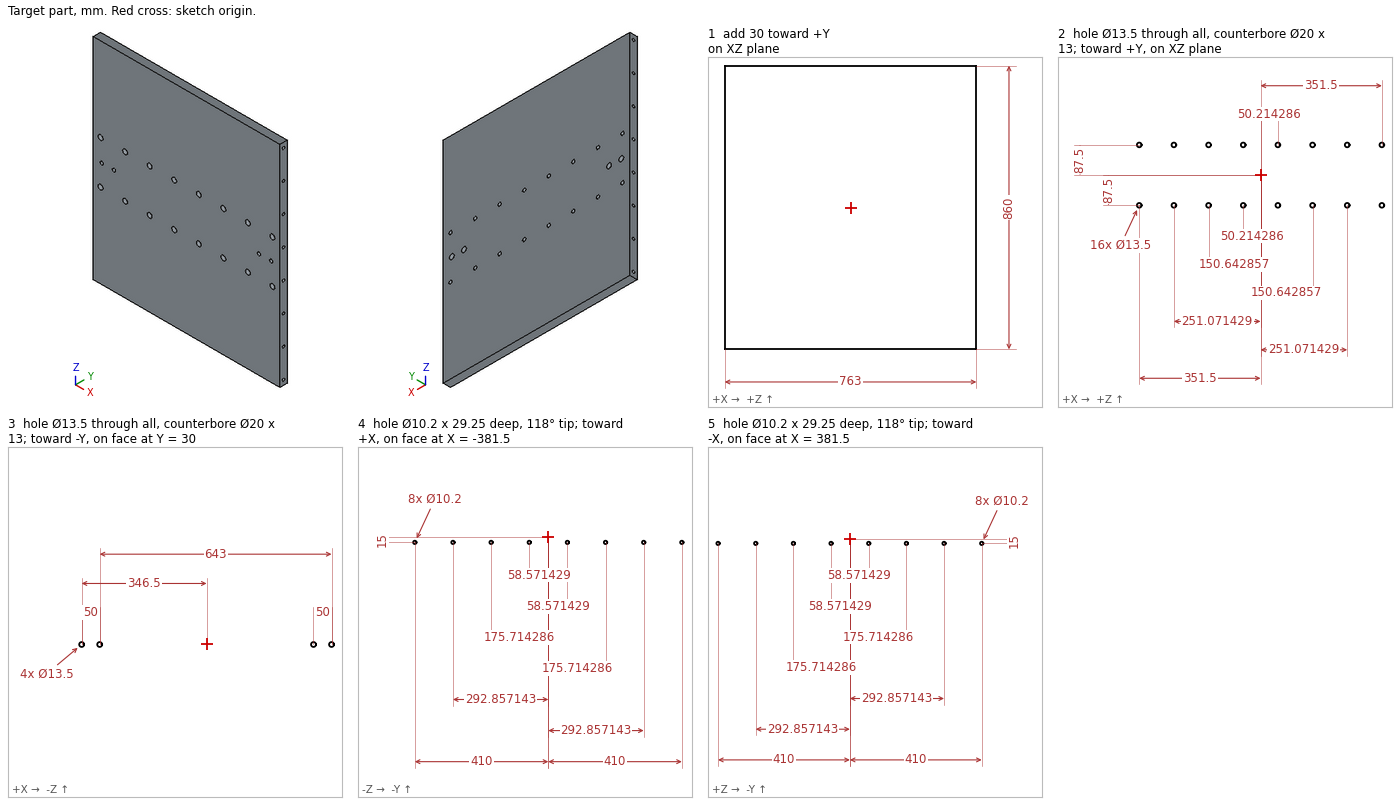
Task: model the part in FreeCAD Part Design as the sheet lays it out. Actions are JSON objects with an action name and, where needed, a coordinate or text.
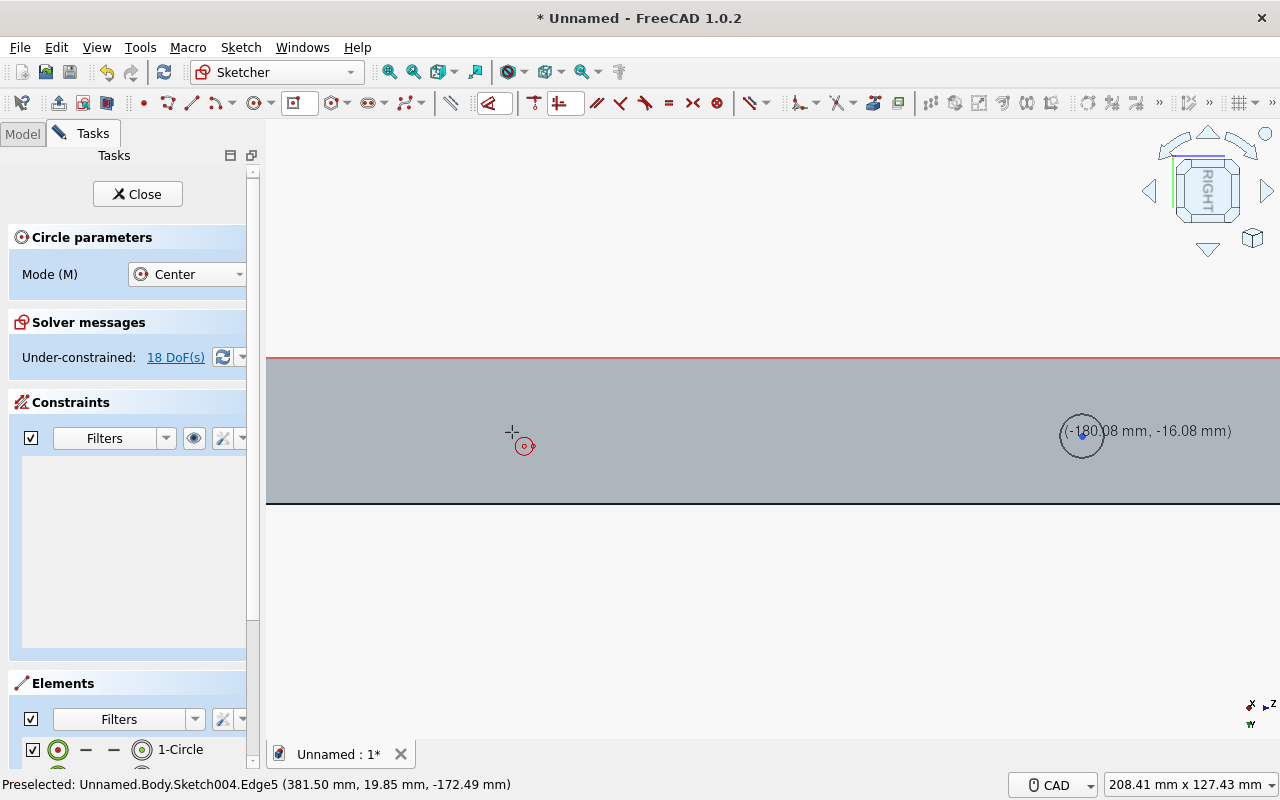
{"action": "scroll", "coordinate": [512, 432], "scroll_direction": "down", "scroll_amount": 10}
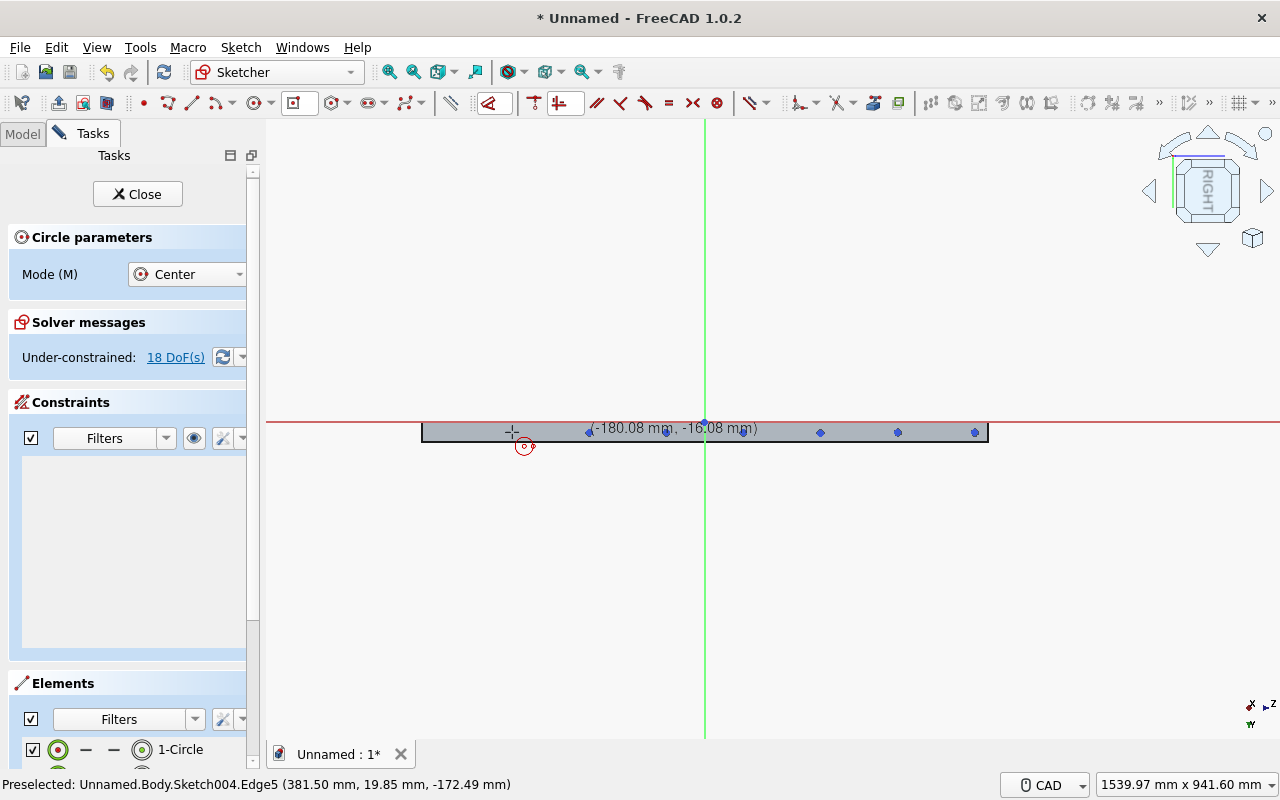
{"action": "scroll", "coordinate": [512, 432], "scroll_direction": "up", "scroll_amount": 3}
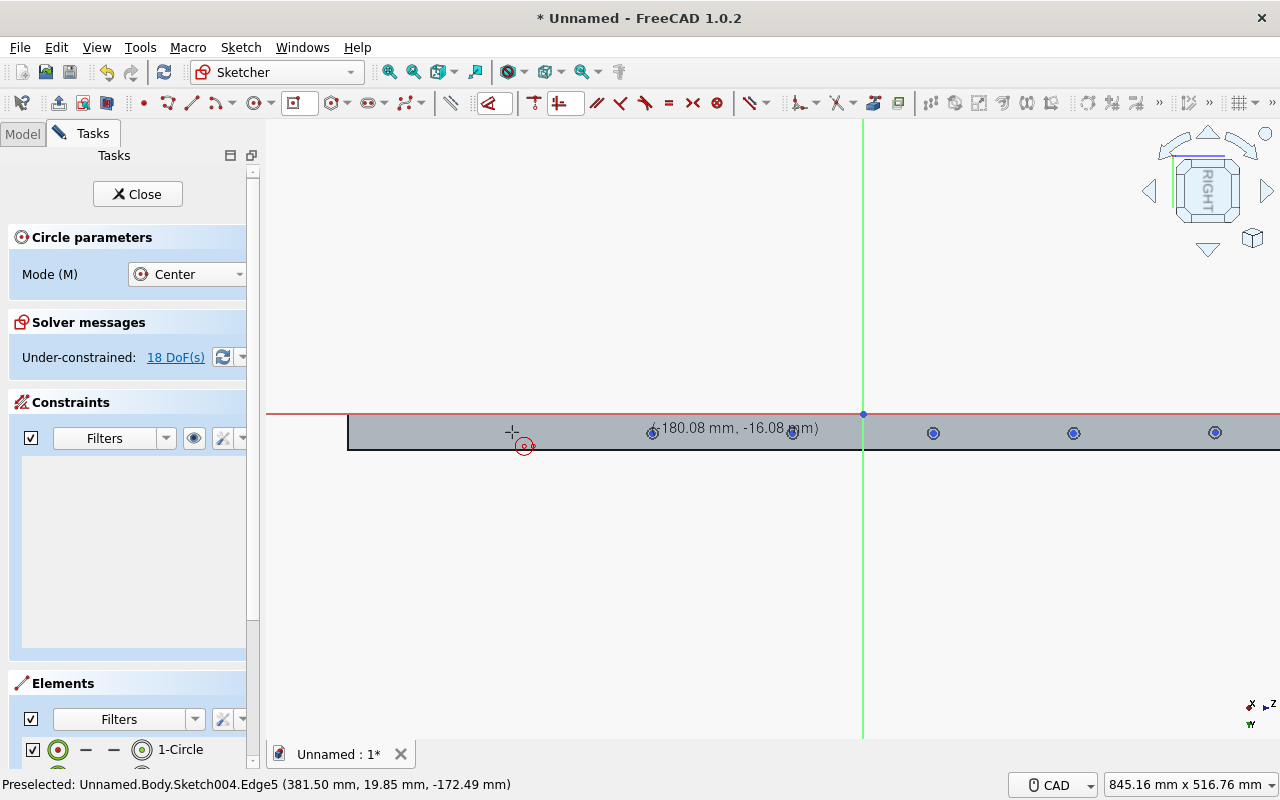
{"action": "left_click", "coordinate": [512, 432]}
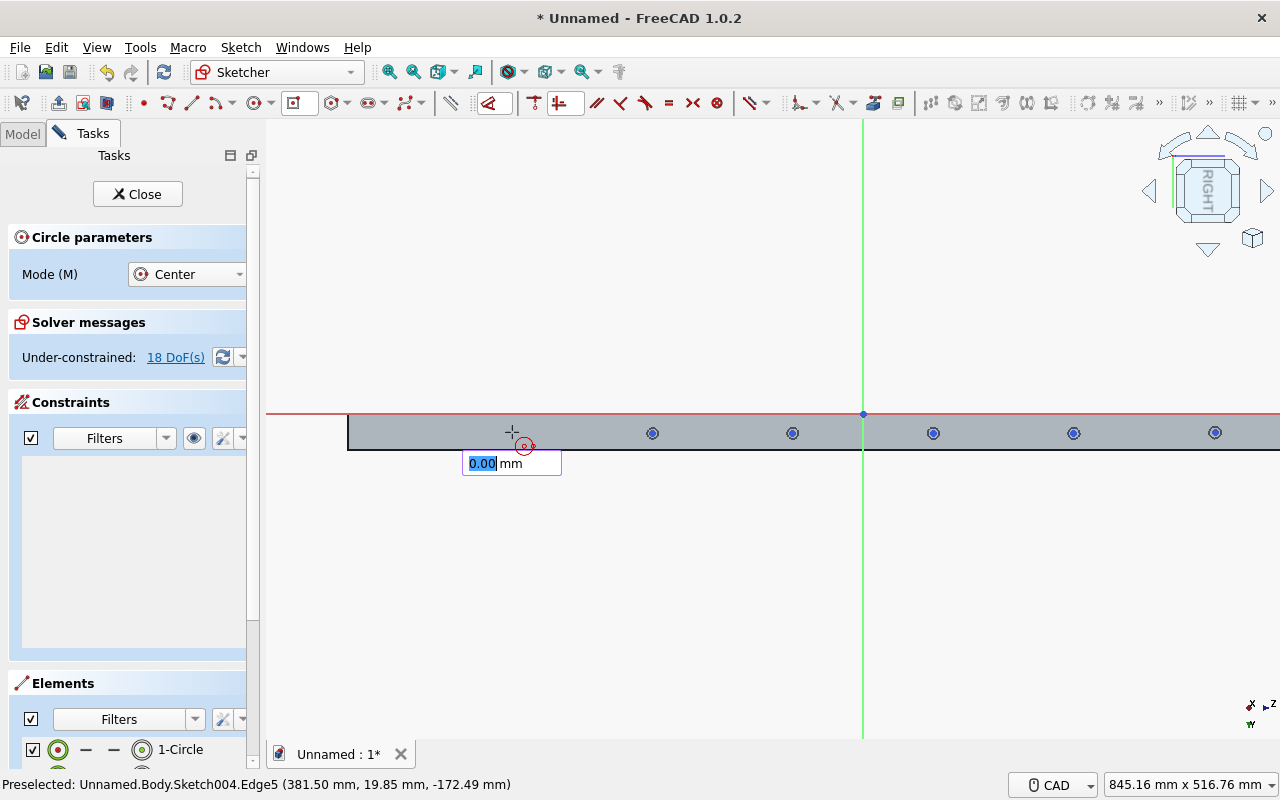
{"action": "scroll", "coordinate": [516, 436], "scroll_direction": "up", "scroll_amount": 5}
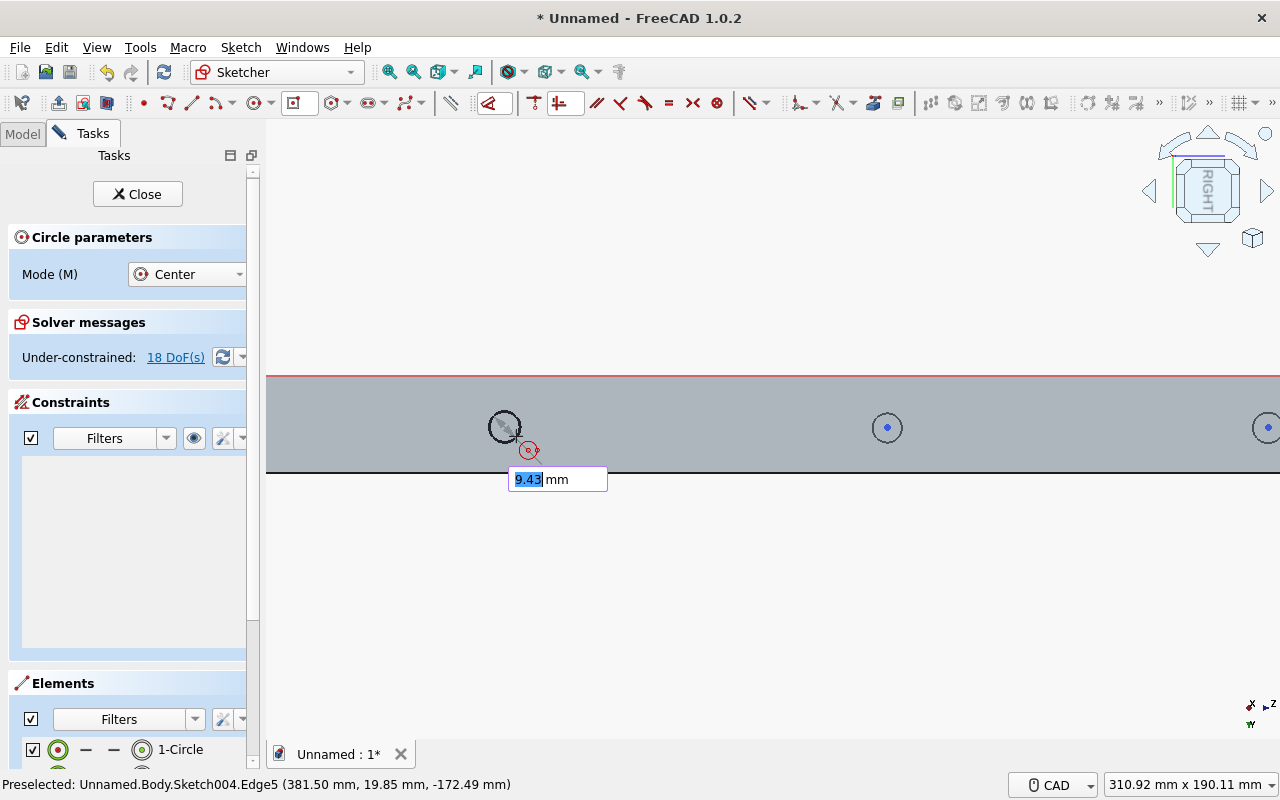
{"action": "left_click", "coordinate": [517, 436]}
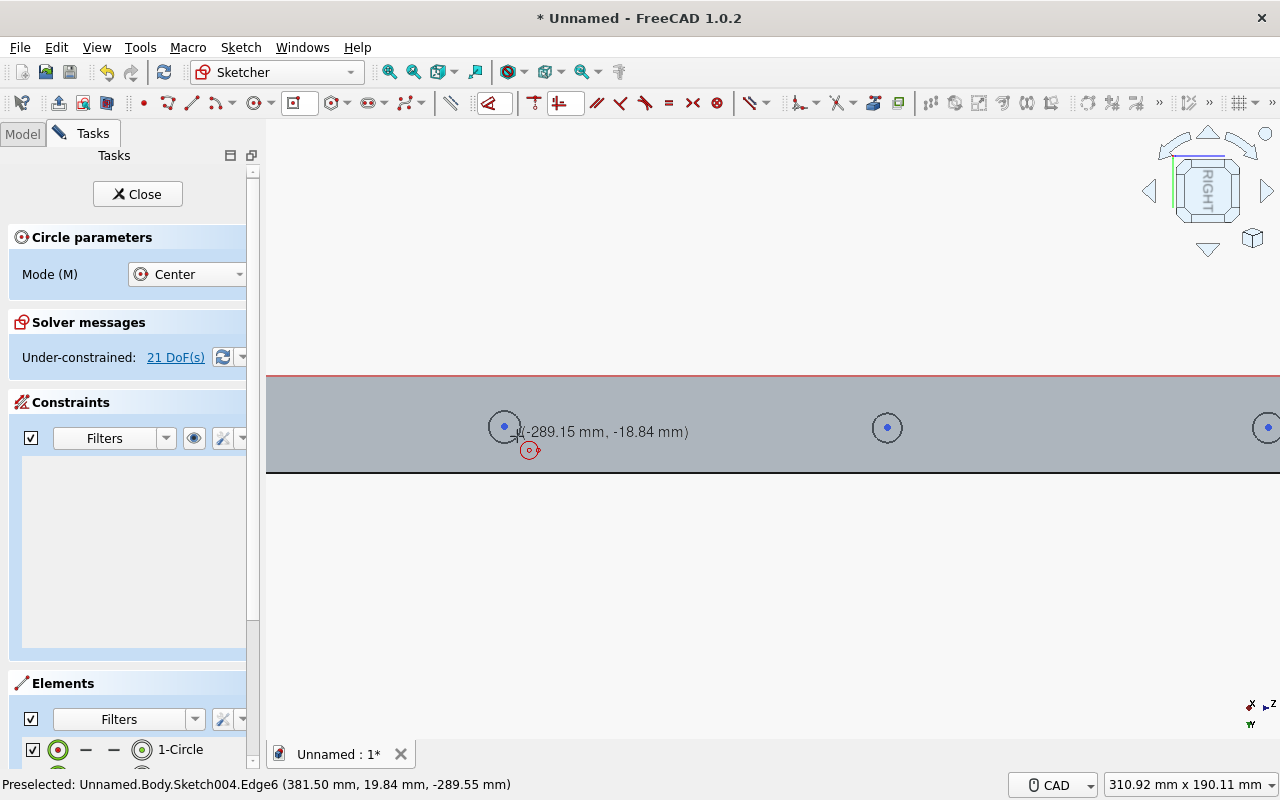
{"action": "scroll", "coordinate": [513, 434], "scroll_direction": "down", "scroll_amount": 8}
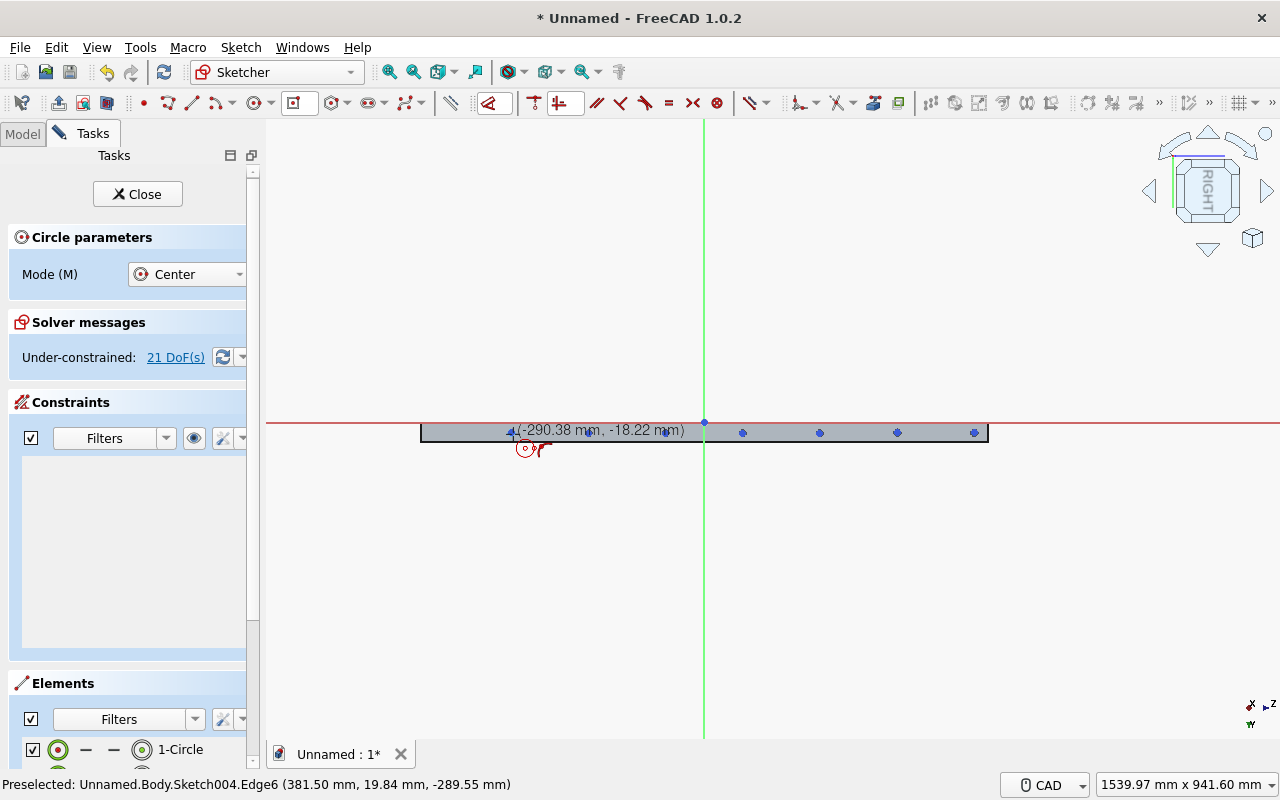
{"action": "scroll", "coordinate": [434, 432], "scroll_direction": "up", "scroll_amount": 10}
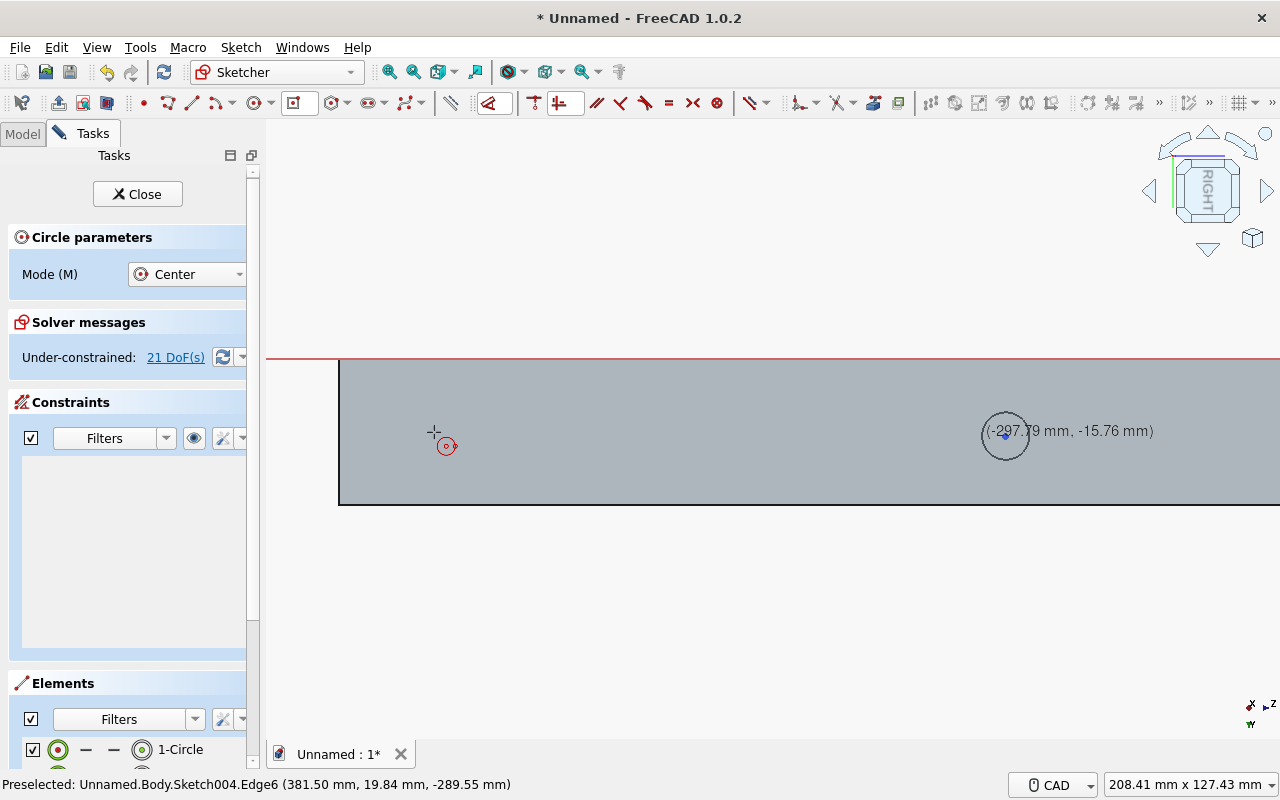
{"action": "scroll", "coordinate": [434, 432], "scroll_direction": "down", "scroll_amount": 10}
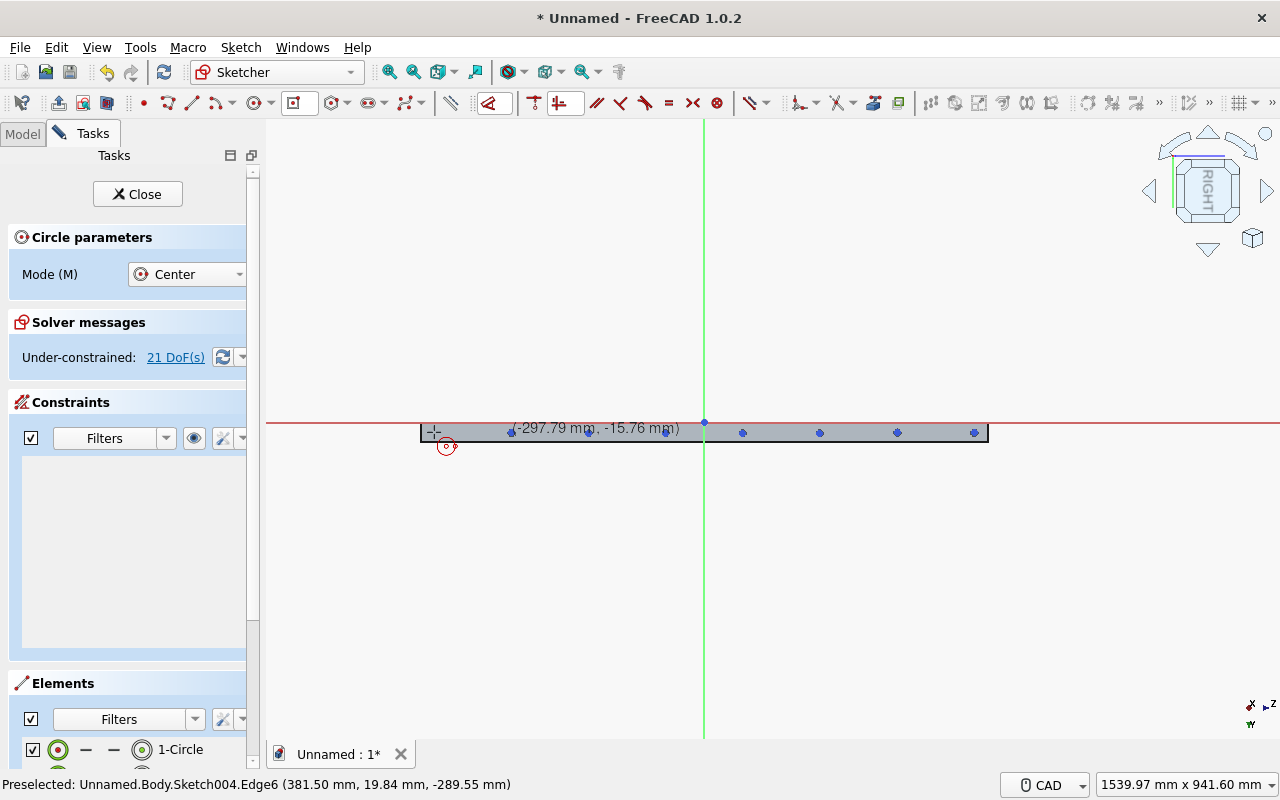
{"action": "scroll", "coordinate": [434, 432], "scroll_direction": "up", "scroll_amount": 3}